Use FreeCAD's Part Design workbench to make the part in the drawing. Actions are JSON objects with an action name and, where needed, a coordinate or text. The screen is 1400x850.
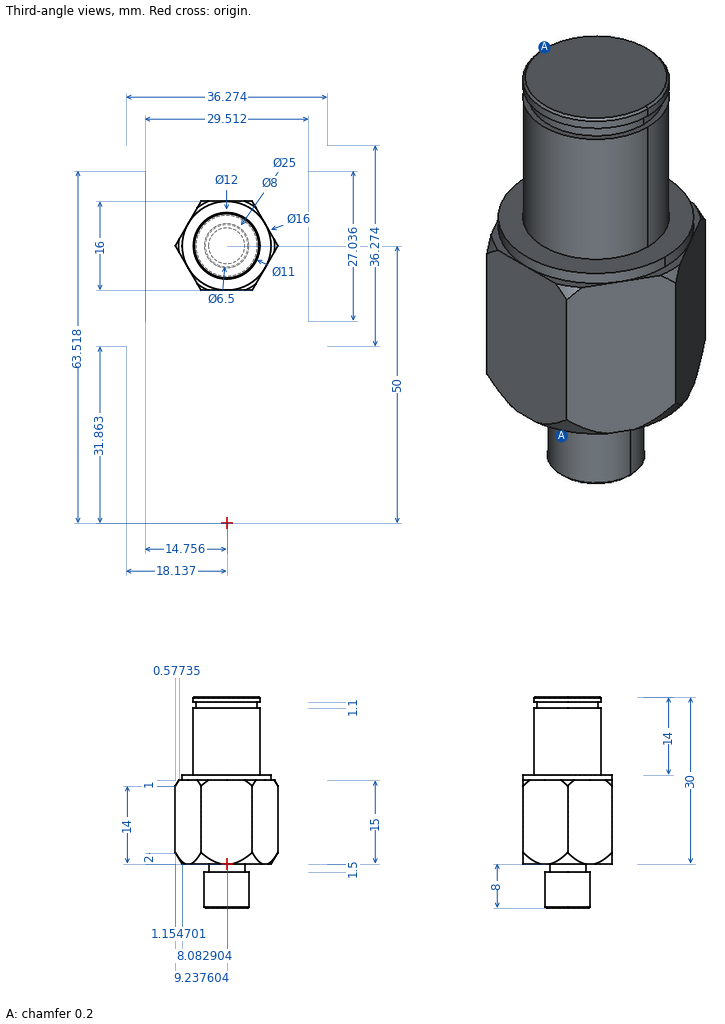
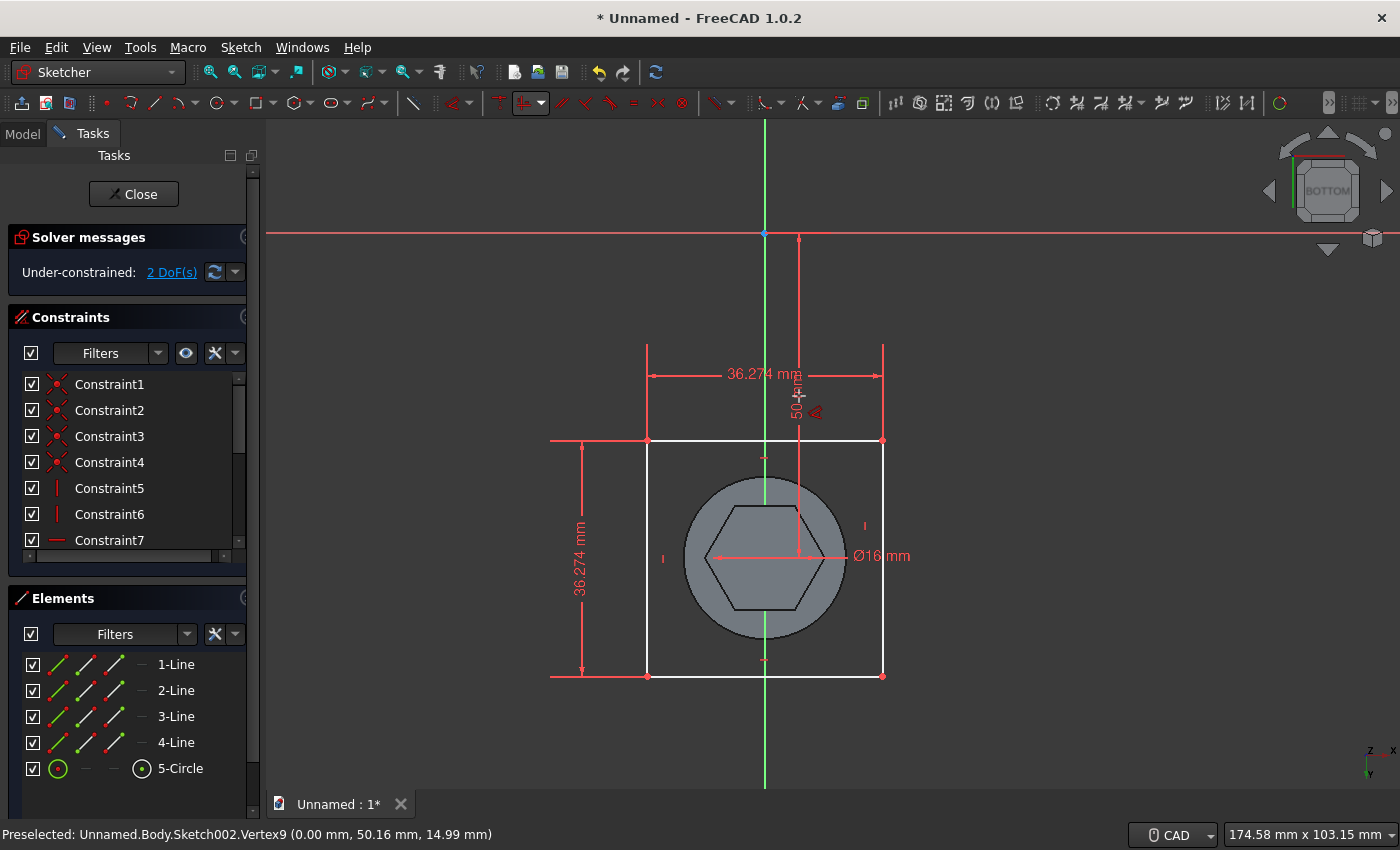
{"action": "left_click", "coordinate": [647, 441]}
{"action": "left_click", "coordinate": [706, 199]}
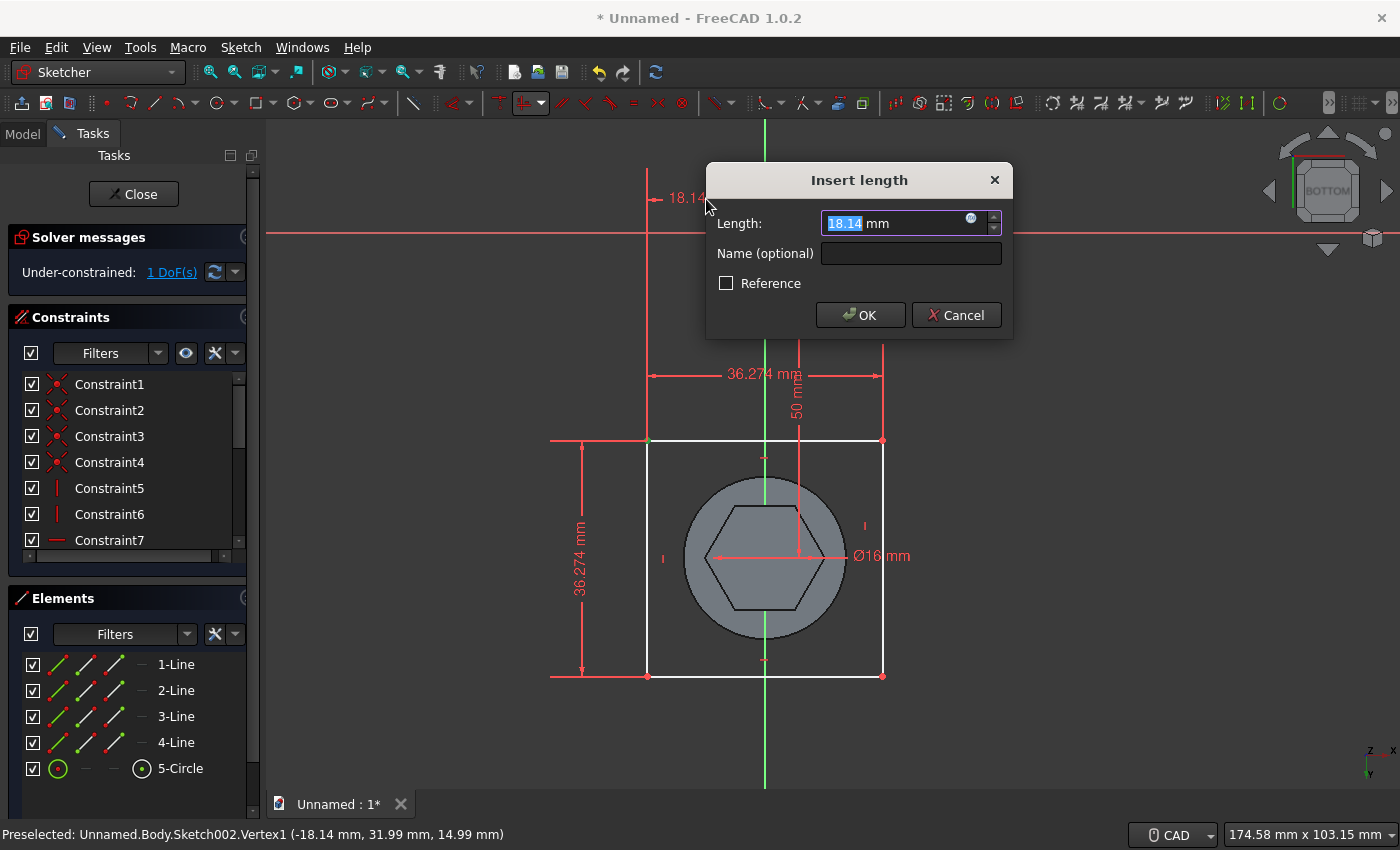
{"action": "type", "text": "18.137"}
{"action": "key", "text": "Return"}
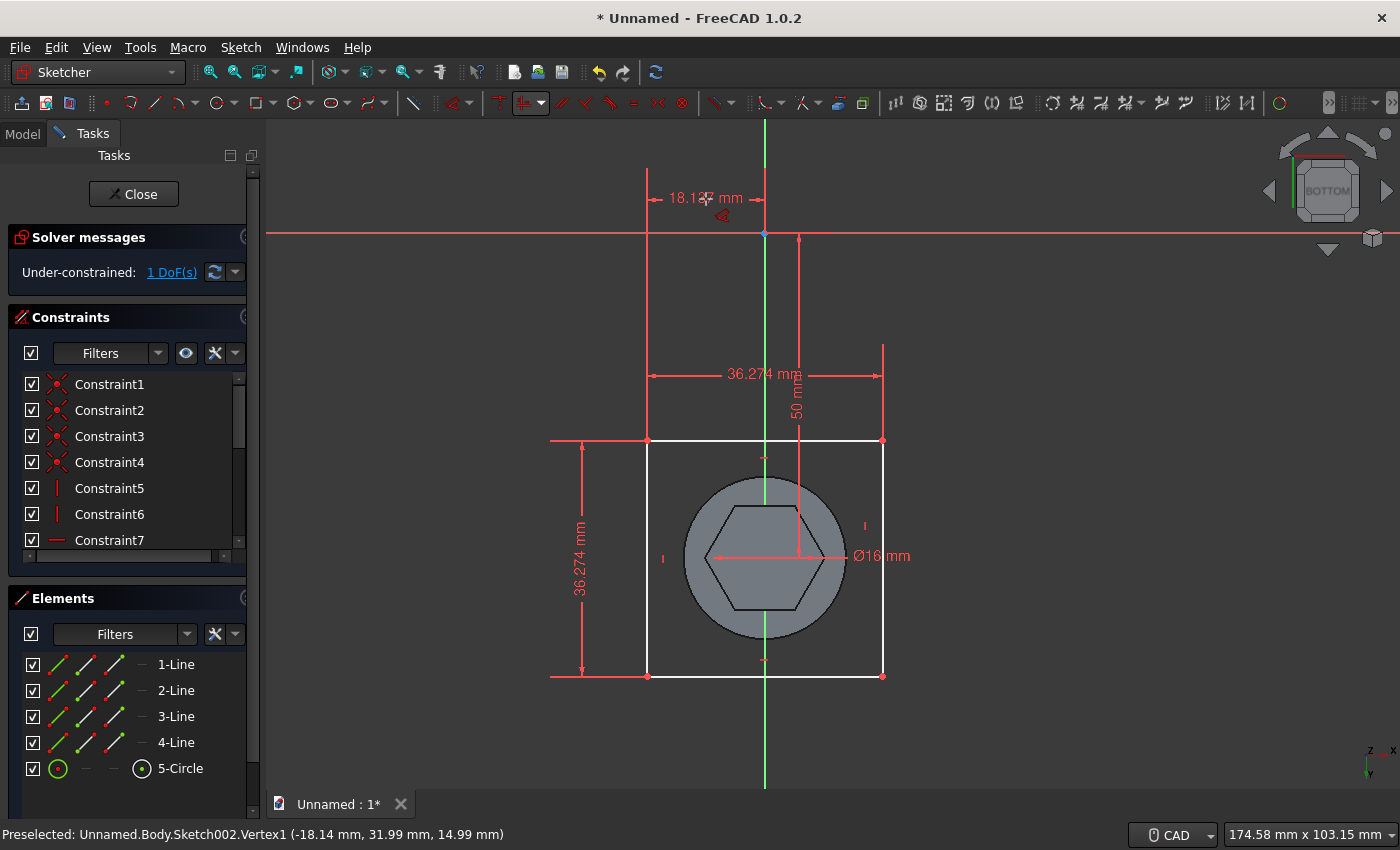
{"action": "left_click", "coordinate": [647, 441]}
{"action": "left_click", "coordinate": [613, 337]}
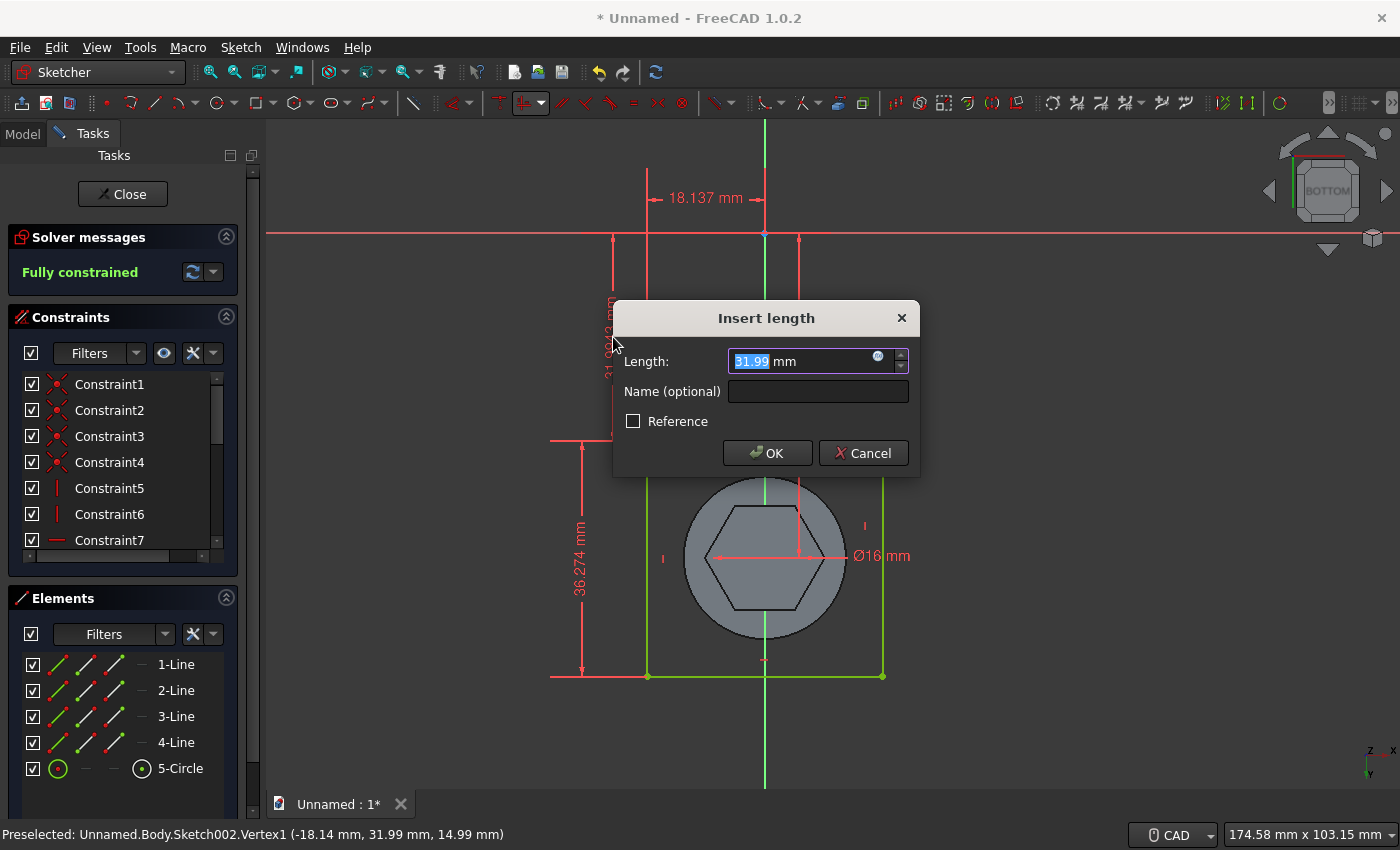
{"action": "type", "text": "31.863"}
{"action": "key", "text": "Return"}
{"action": "key", "text": "Escape"}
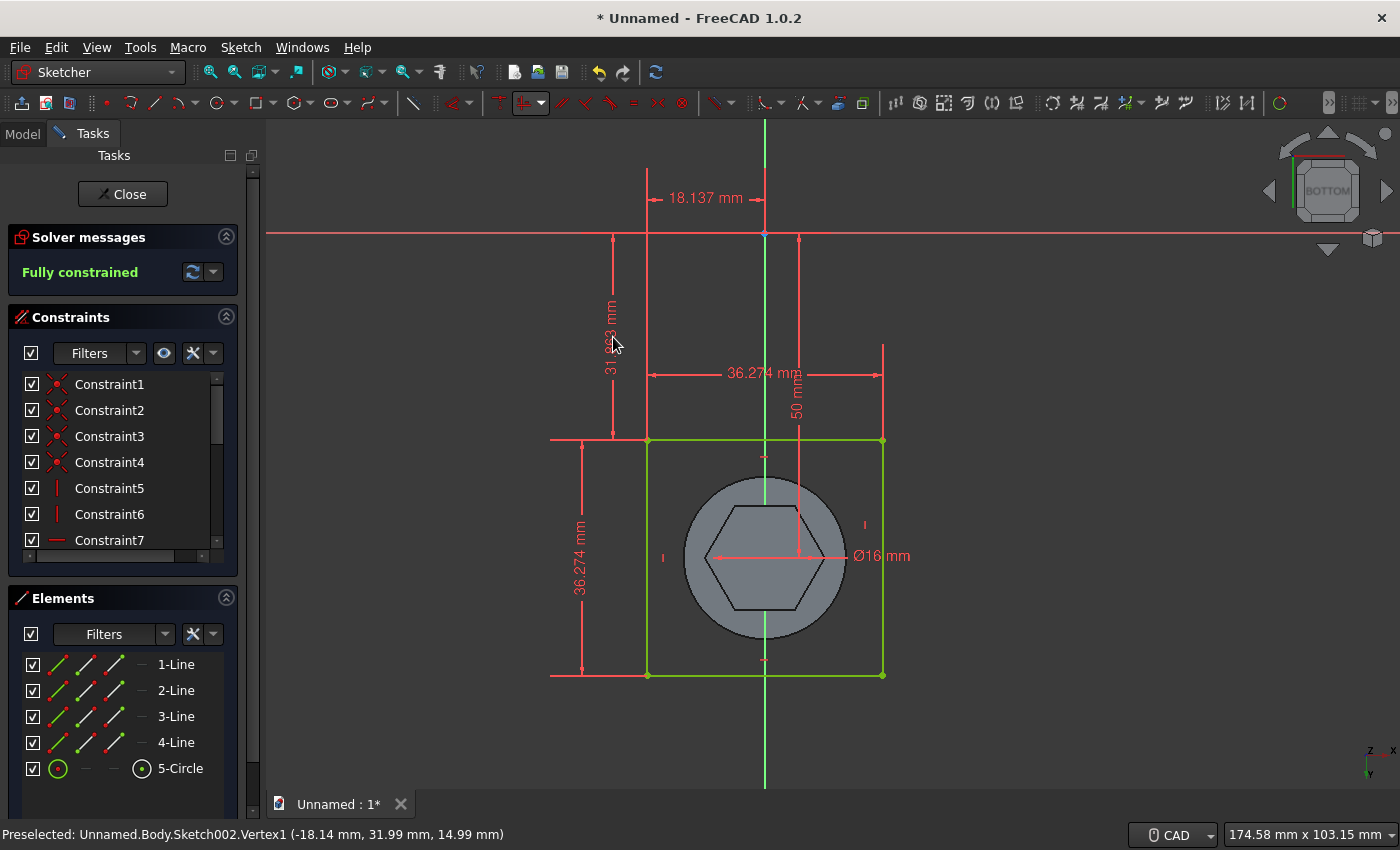
{"action": "left_click", "coordinate": [123, 194]}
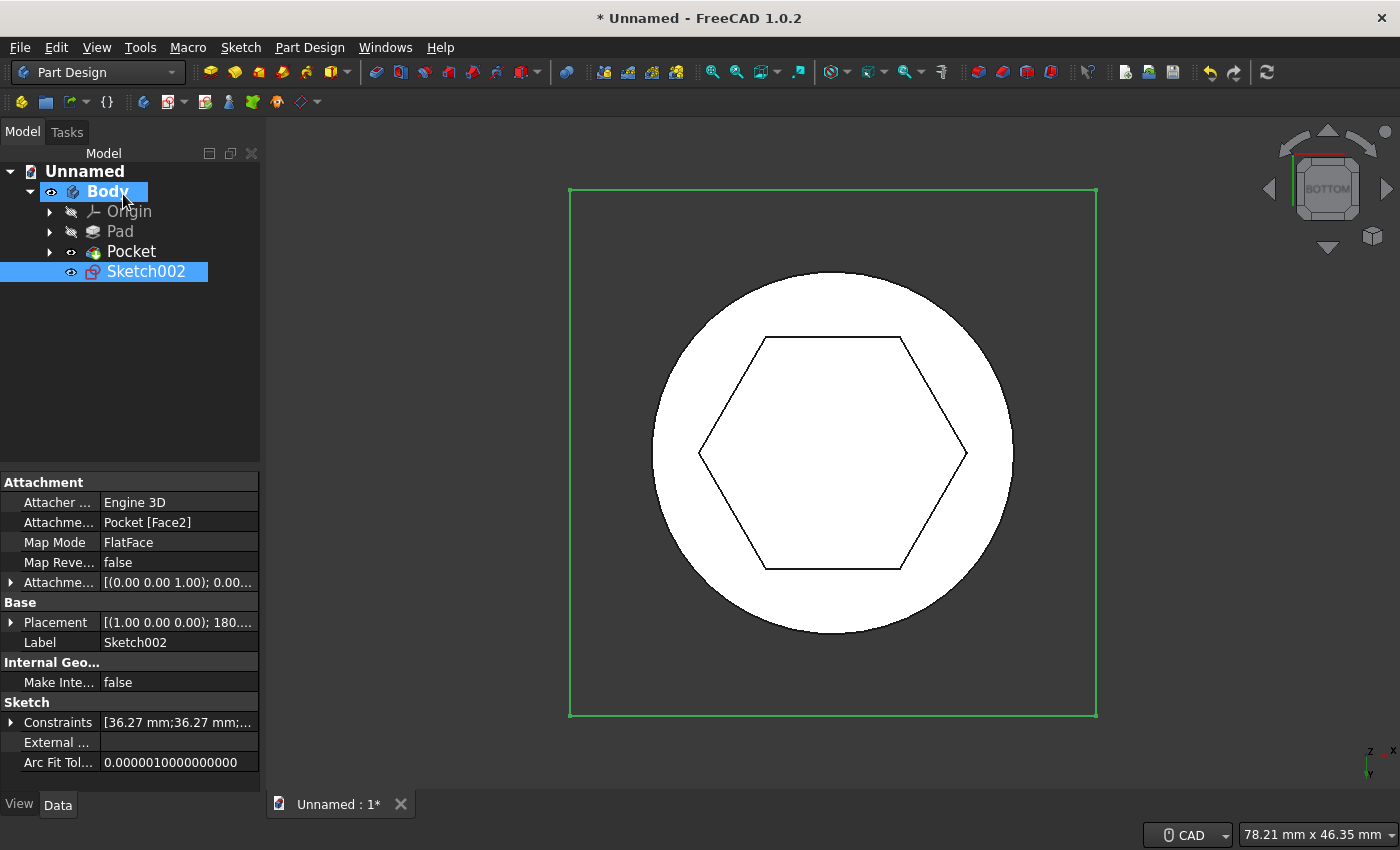
{"action": "left_click", "coordinate": [378, 72]}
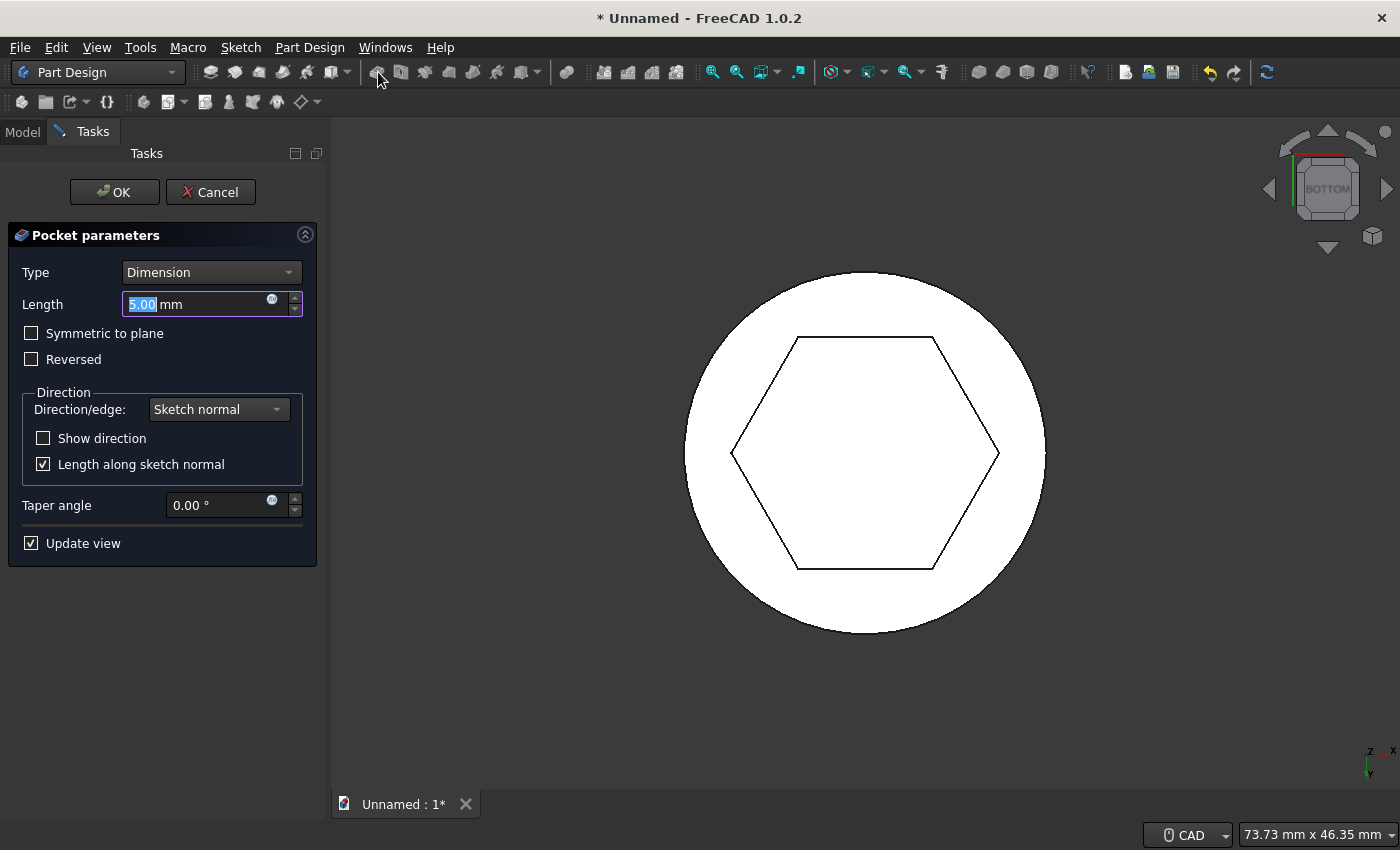
{"action": "left_click", "coordinate": [212, 272]}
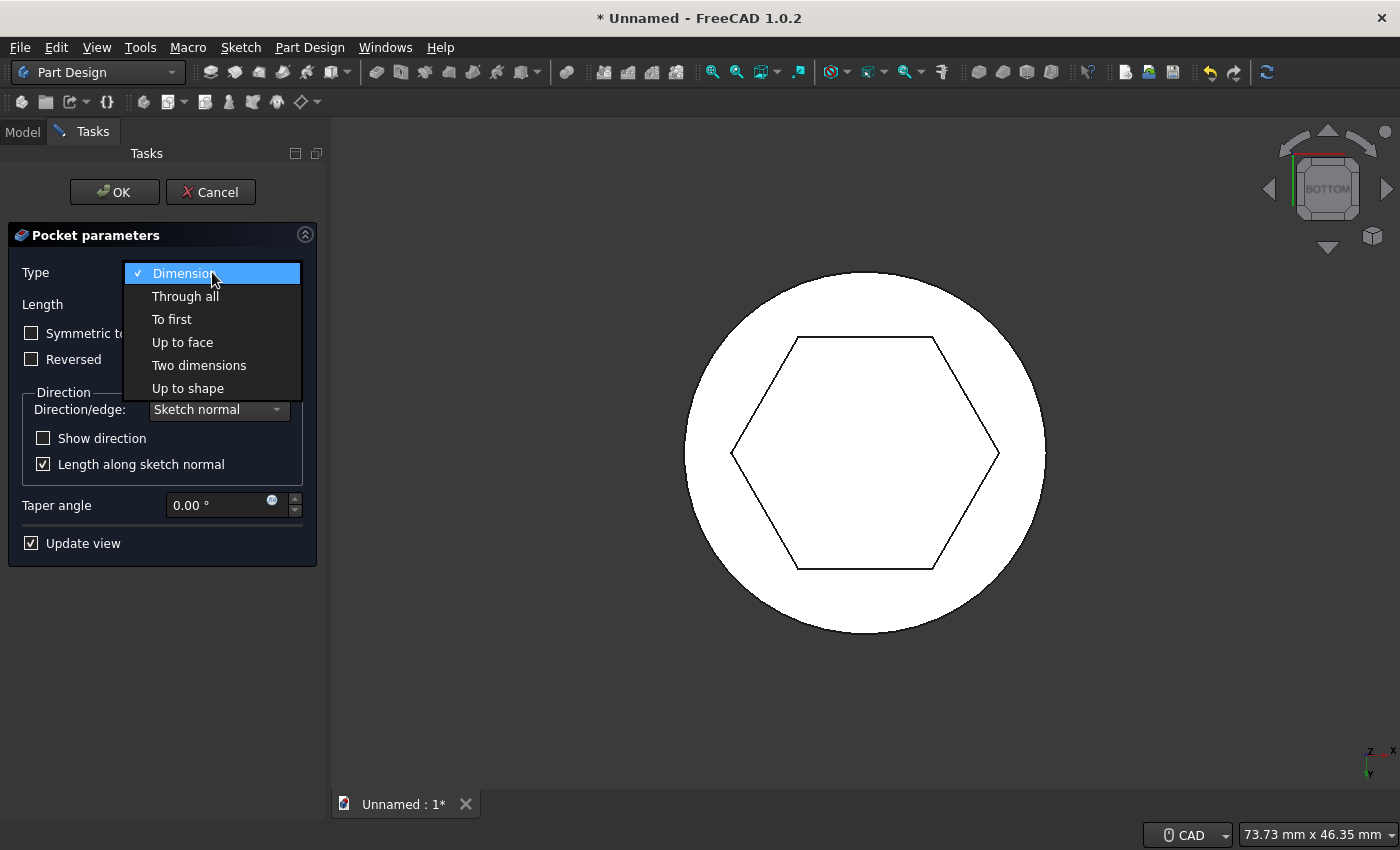
{"action": "left_click", "coordinate": [212, 296]}